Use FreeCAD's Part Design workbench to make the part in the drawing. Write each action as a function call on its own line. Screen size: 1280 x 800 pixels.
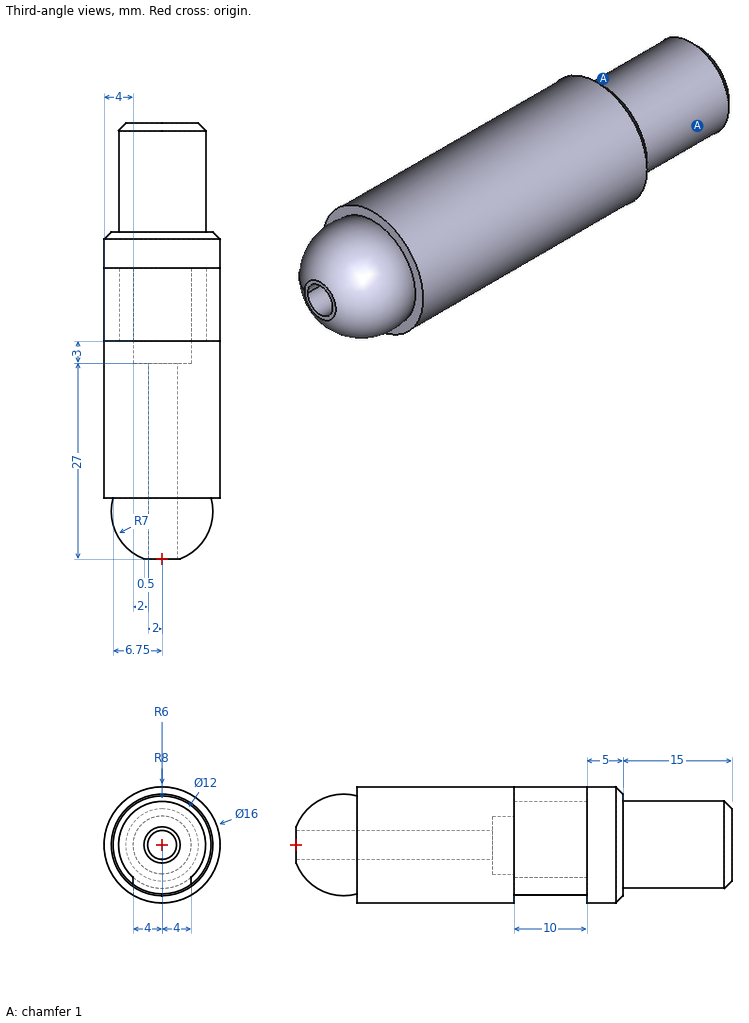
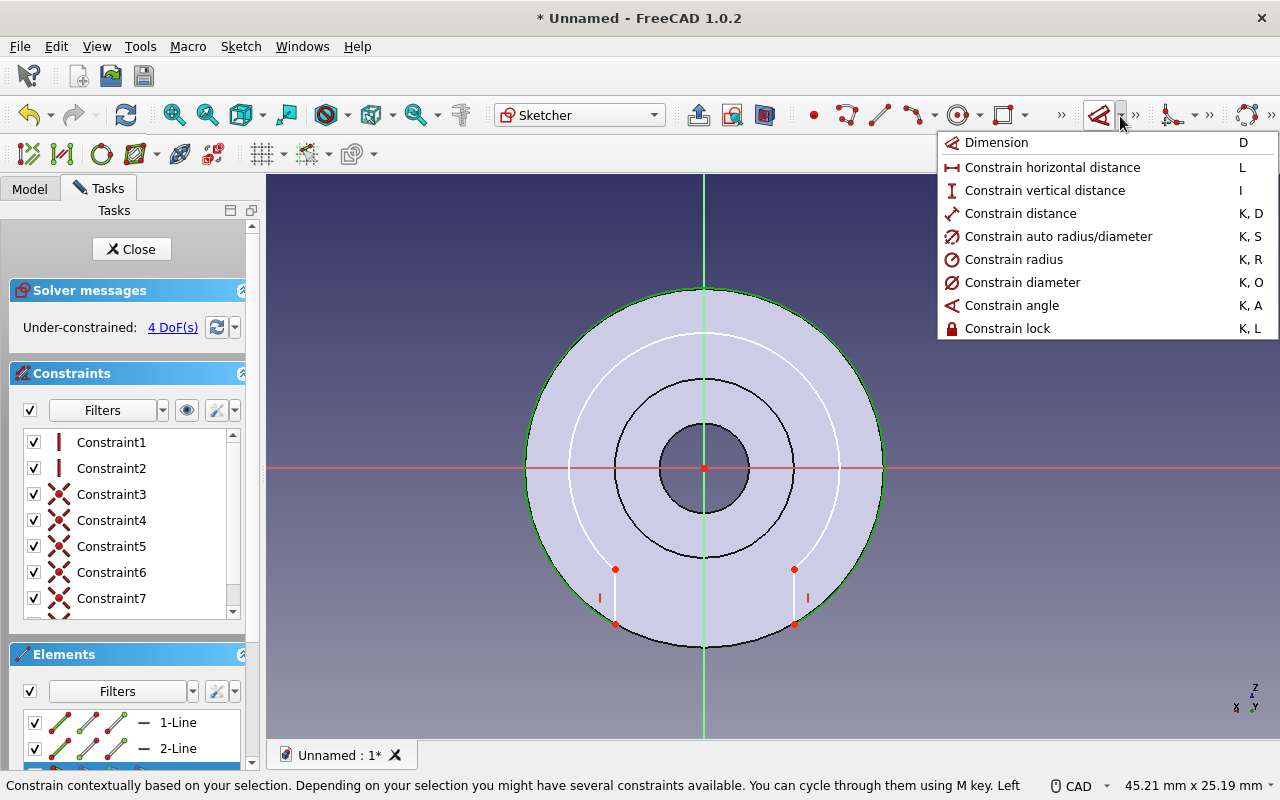
click(1108, 260)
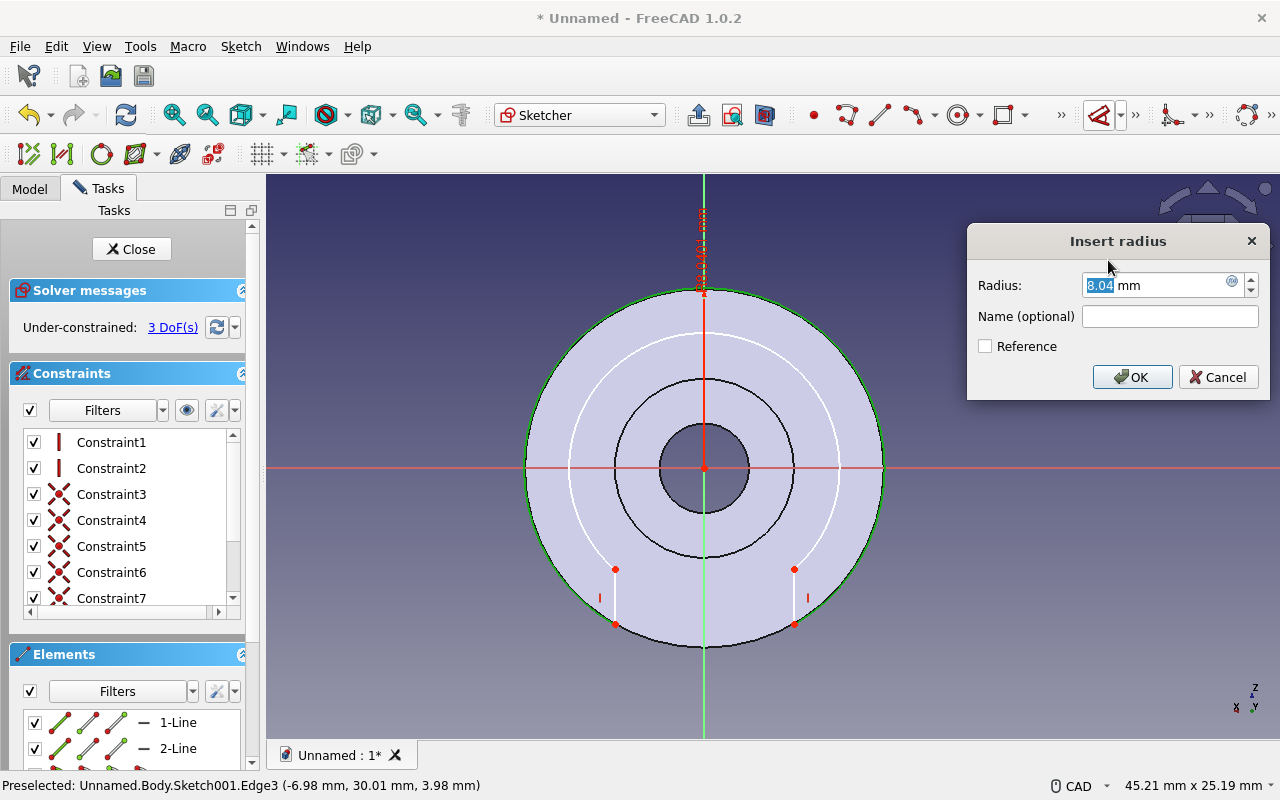
text(8)
key(Return)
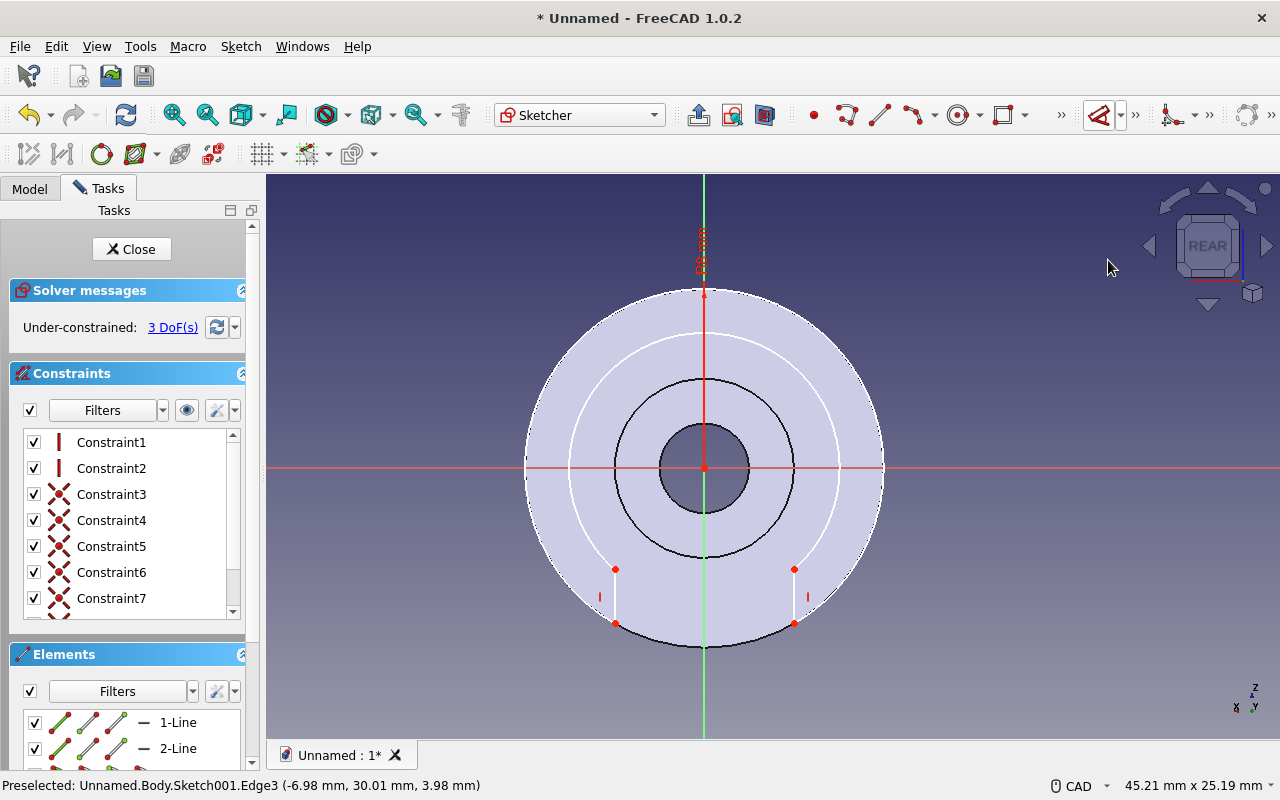
click(816, 391)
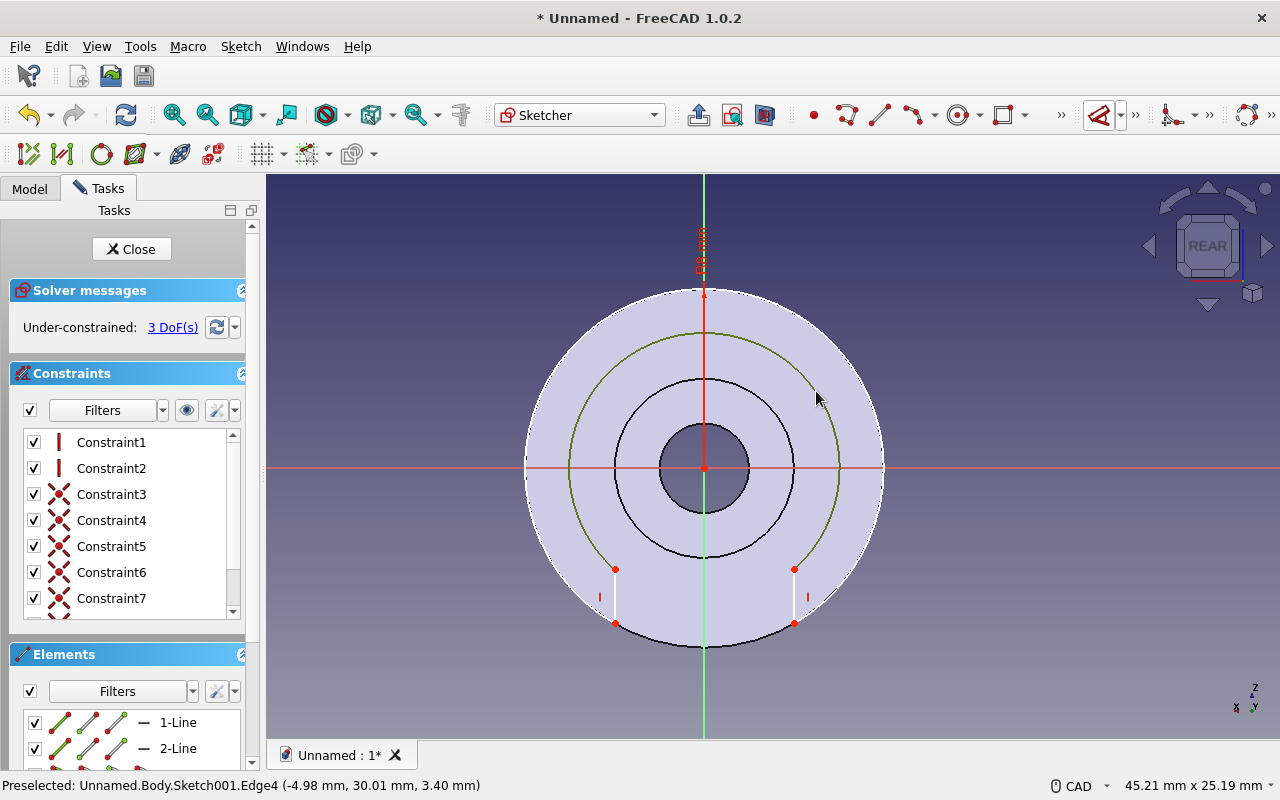
click(1120, 116)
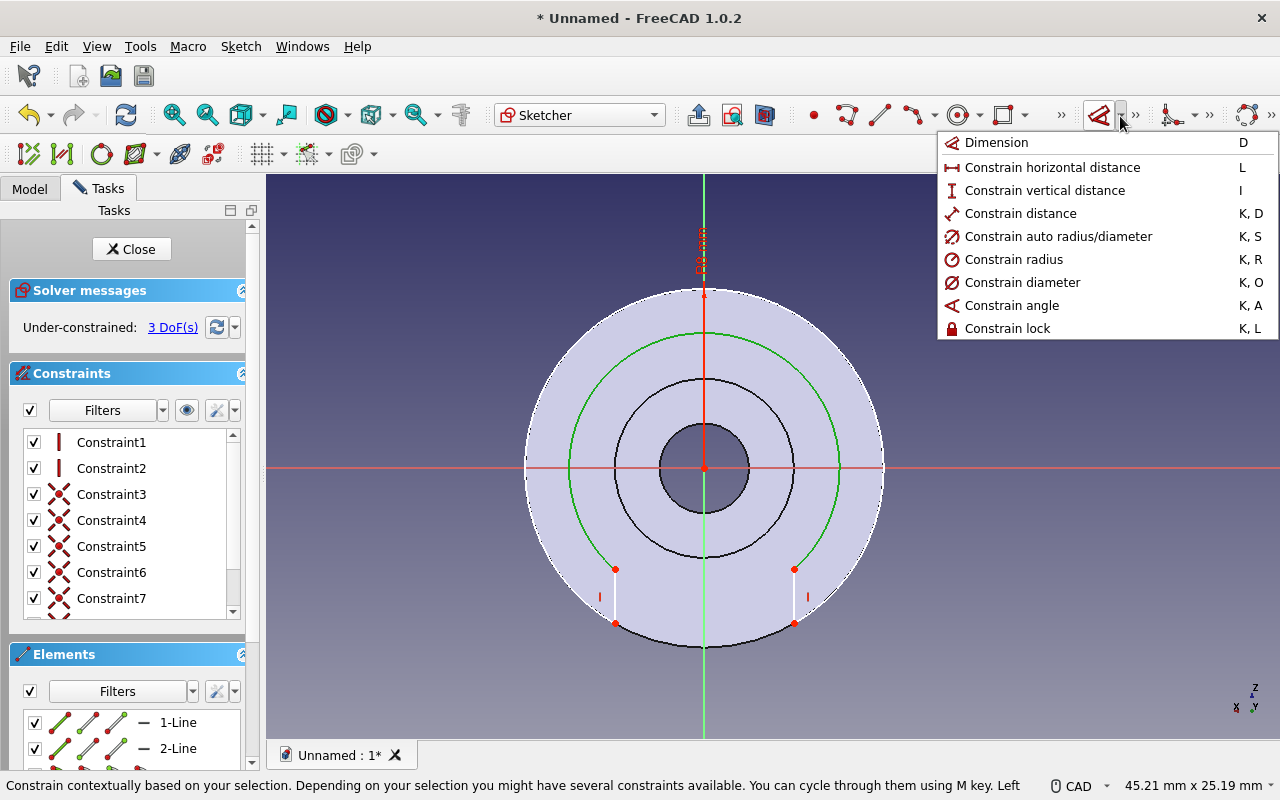
click(1108, 260)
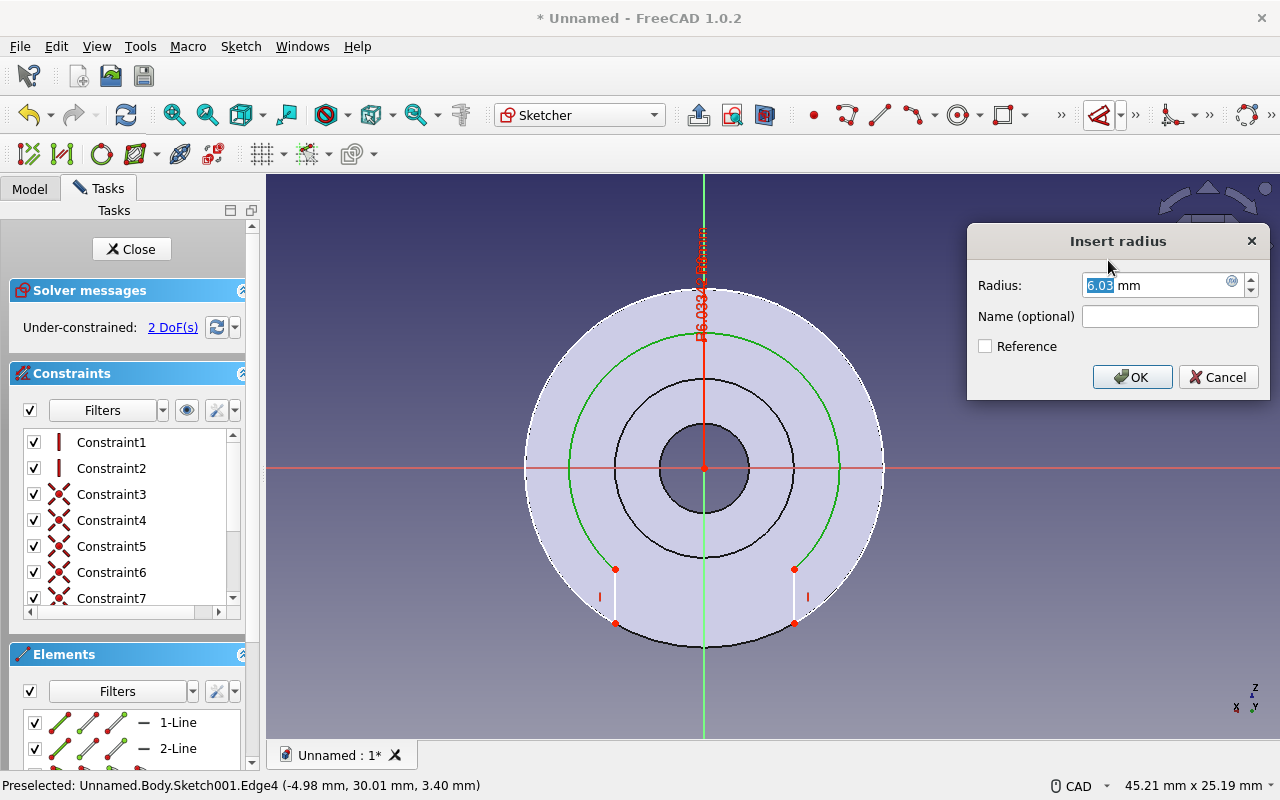
text(6)
key(Return)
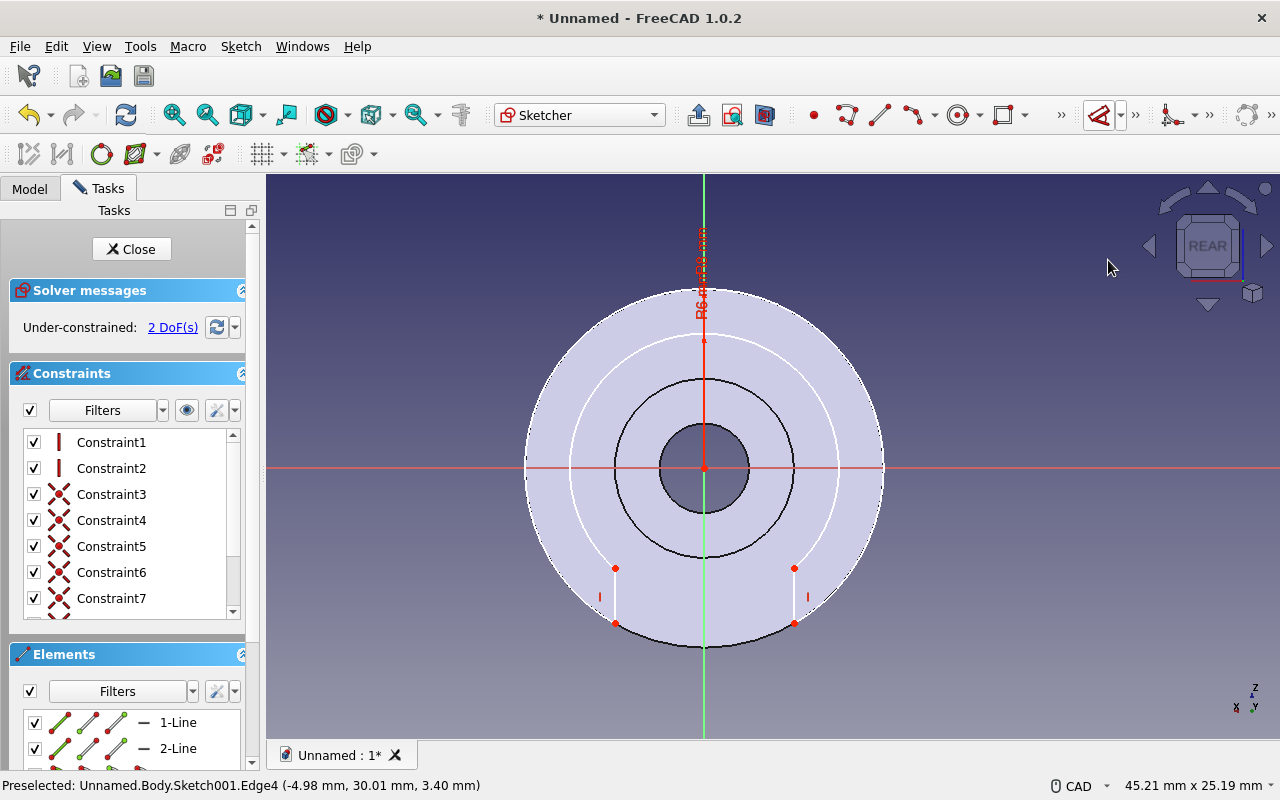
click(794, 569)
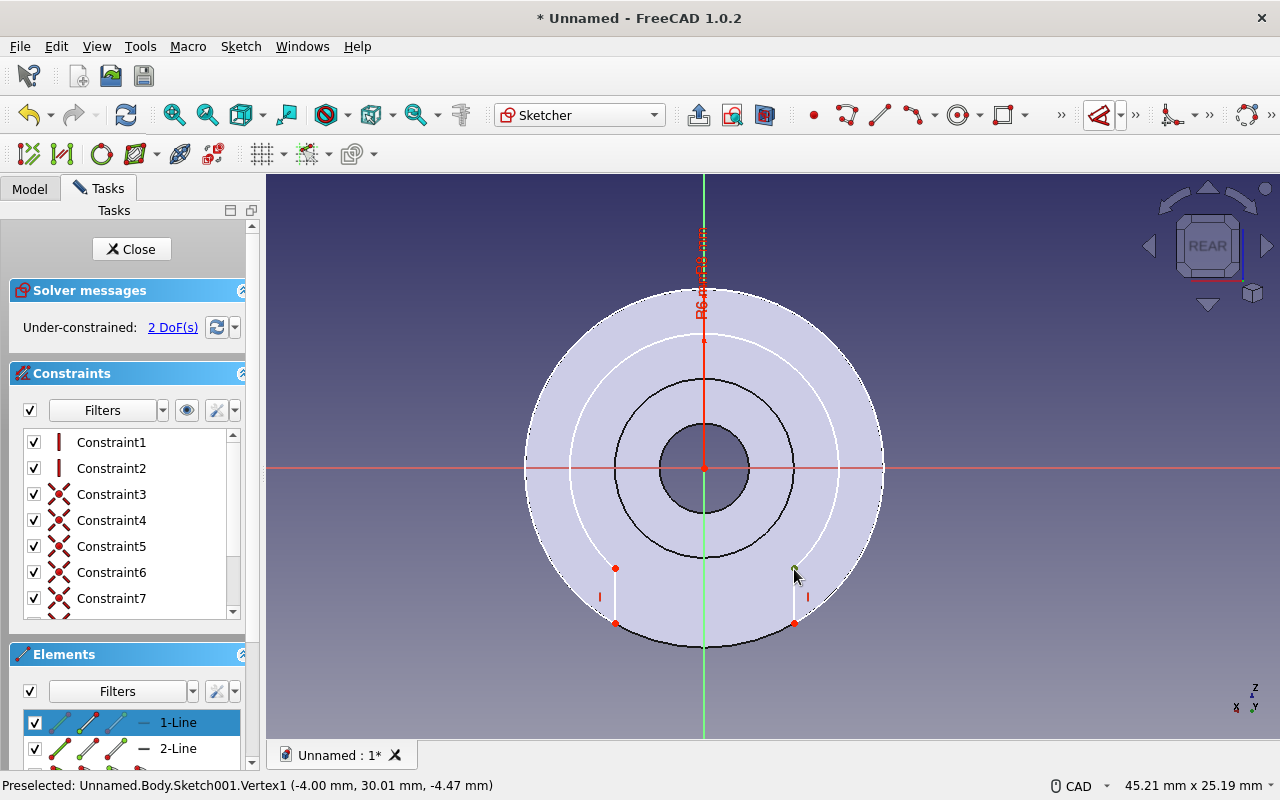
key(l)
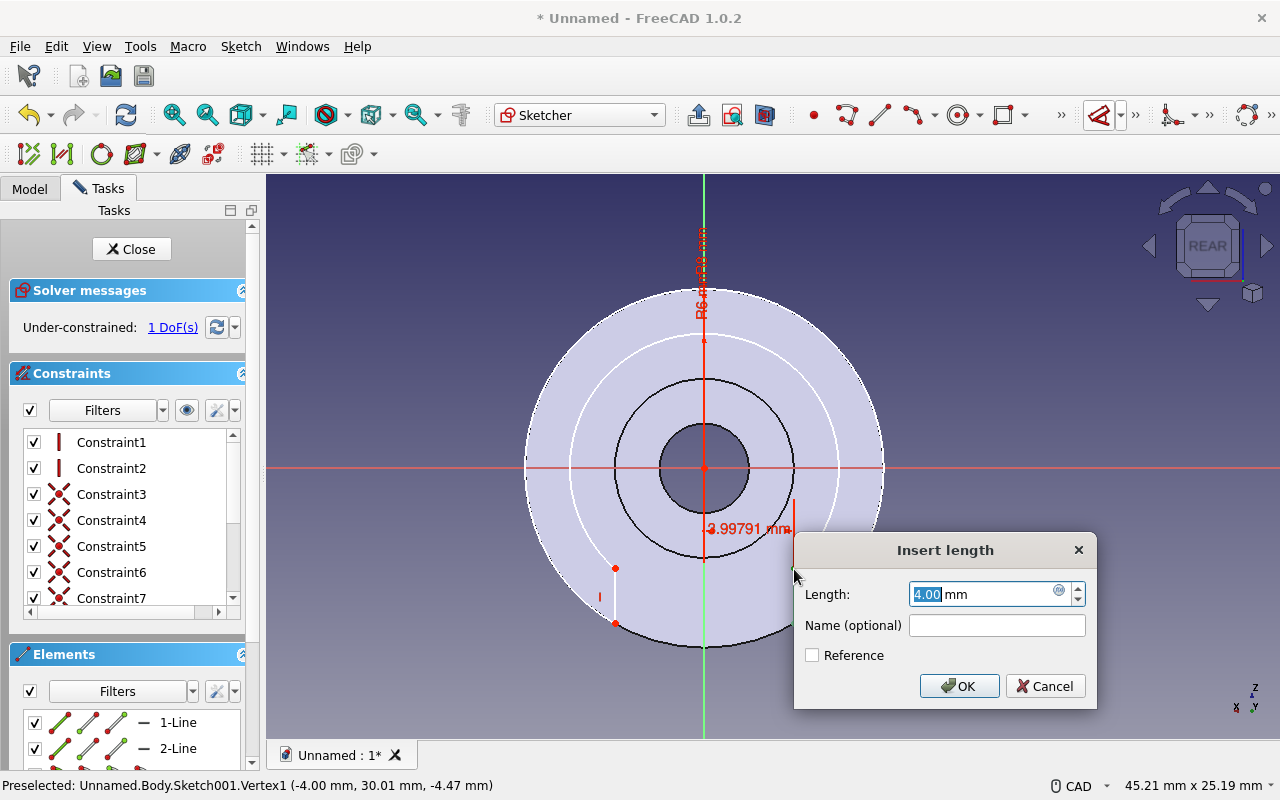
text(4)
key(Return)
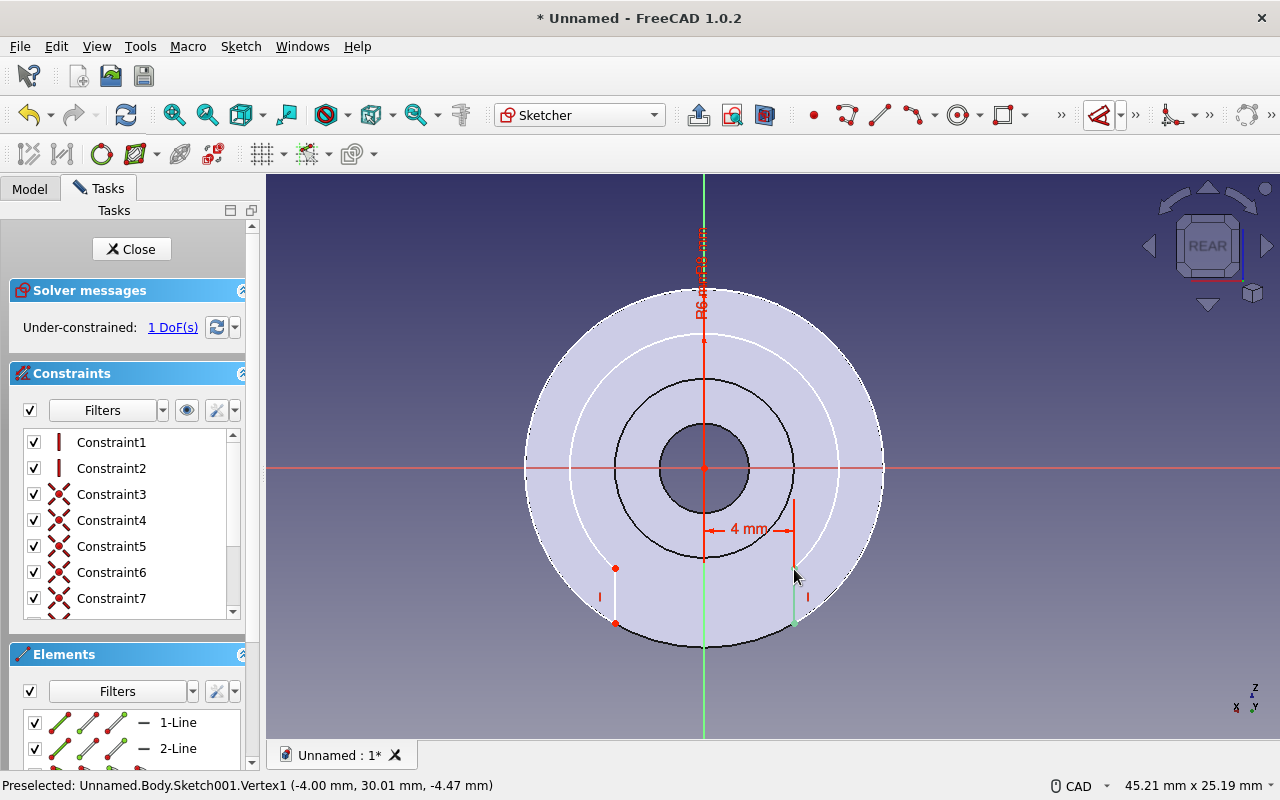
click(615, 624)